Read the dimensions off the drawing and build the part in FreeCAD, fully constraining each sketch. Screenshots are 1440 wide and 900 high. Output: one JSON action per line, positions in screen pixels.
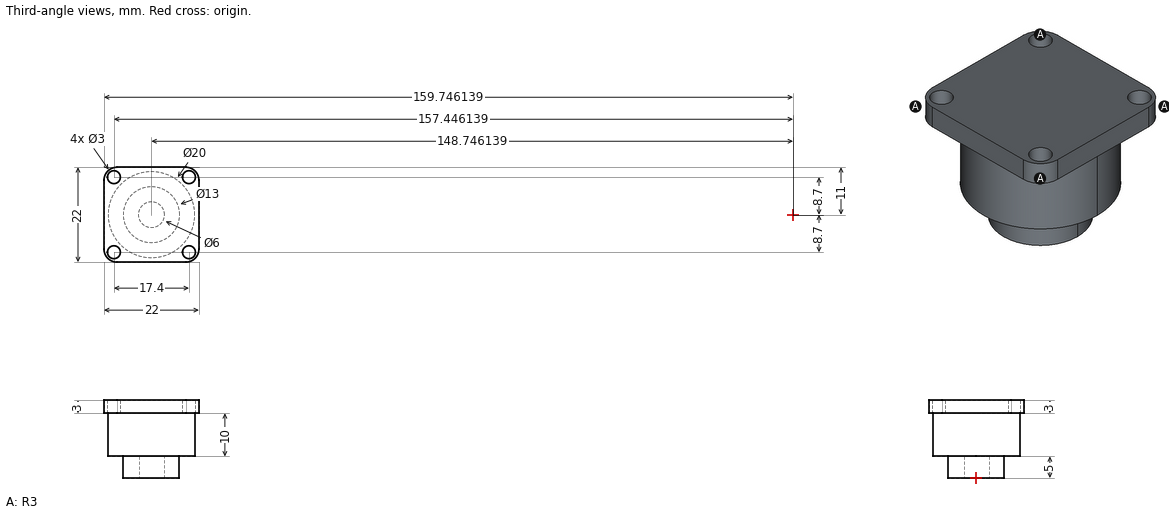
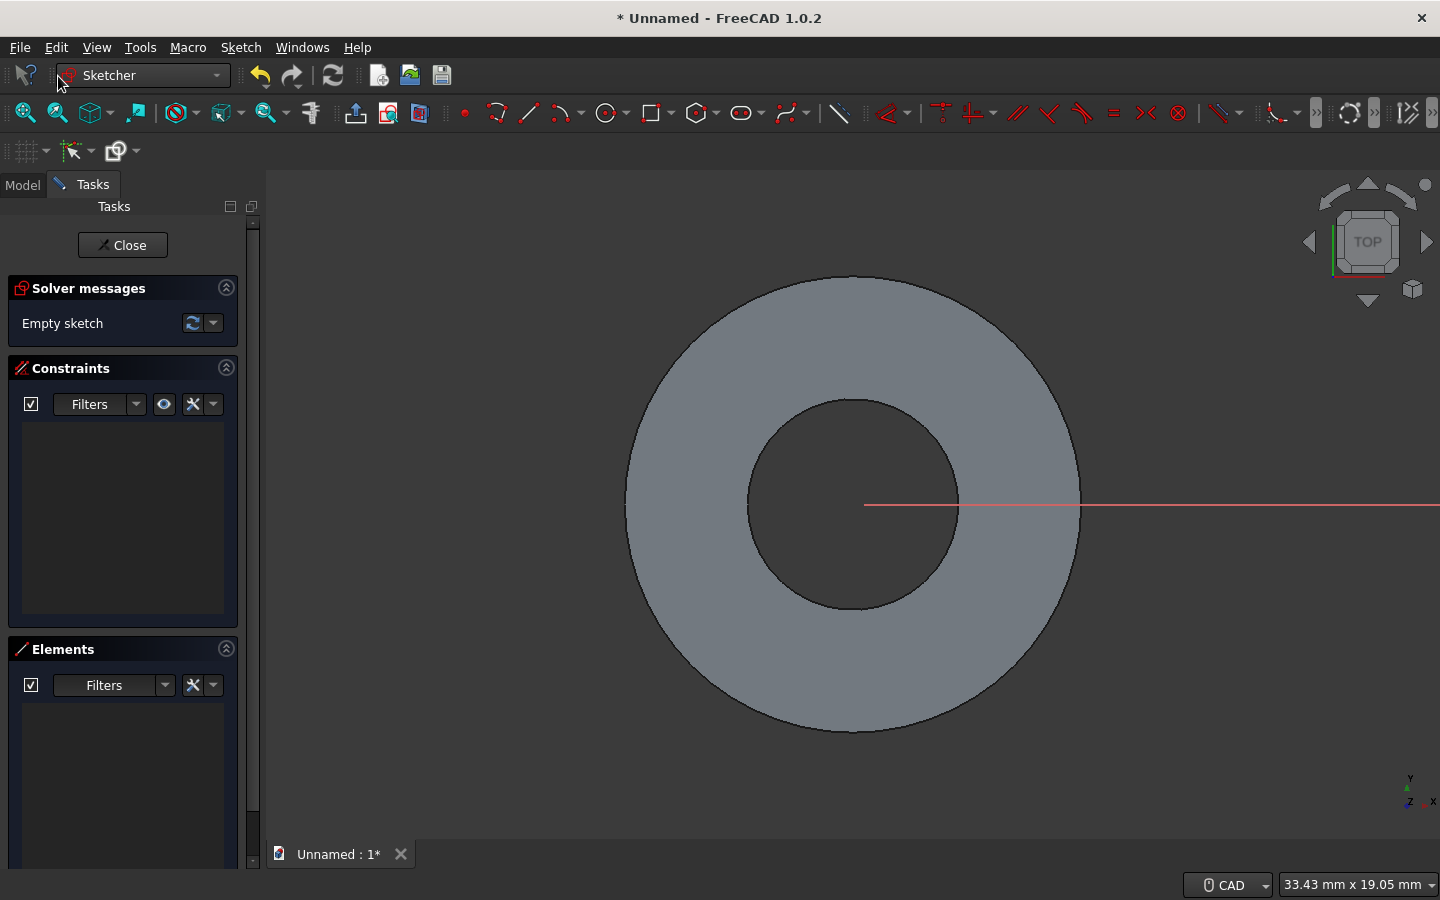
{"action": "scroll", "coordinate": [645, 504], "scroll_direction": "down", "scroll_amount": 2}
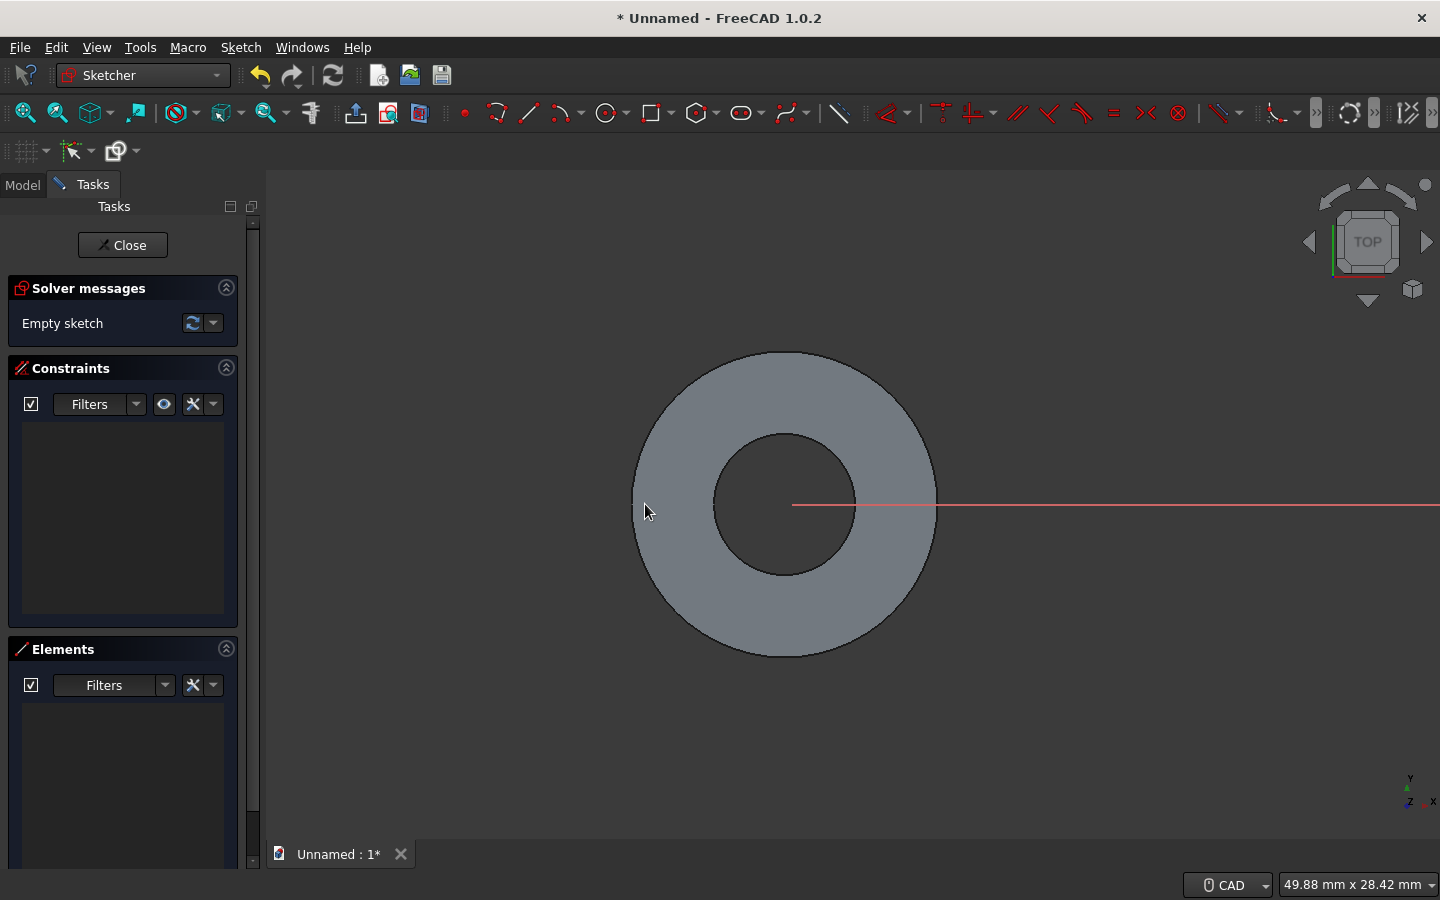
{"action": "left_click", "coordinate": [606, 114]}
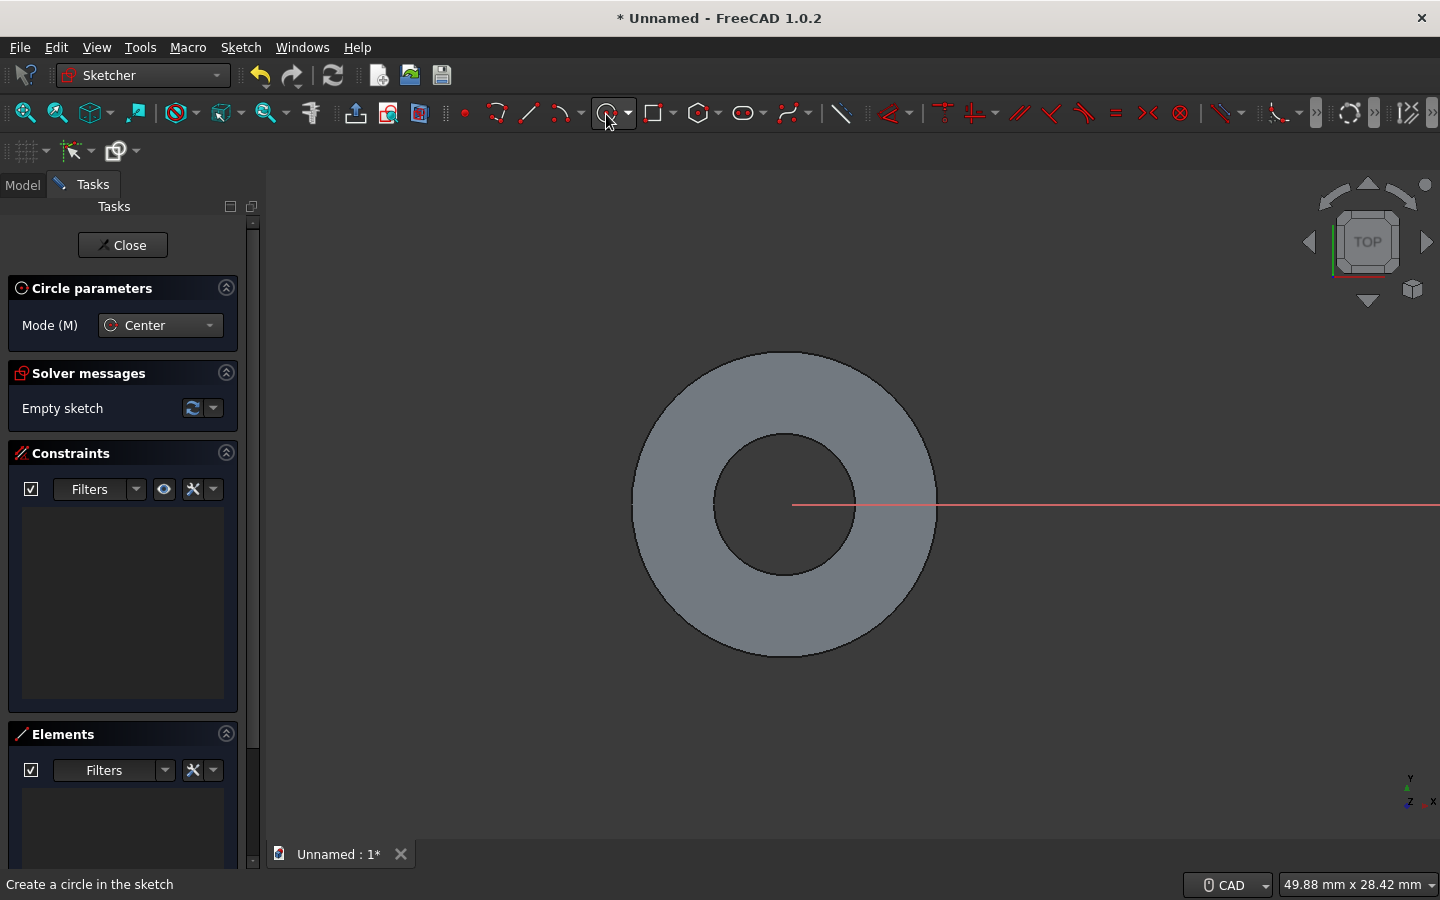
{"action": "left_click", "coordinate": [785, 504]}
{"action": "mouse_move", "coordinate": [951, 338]}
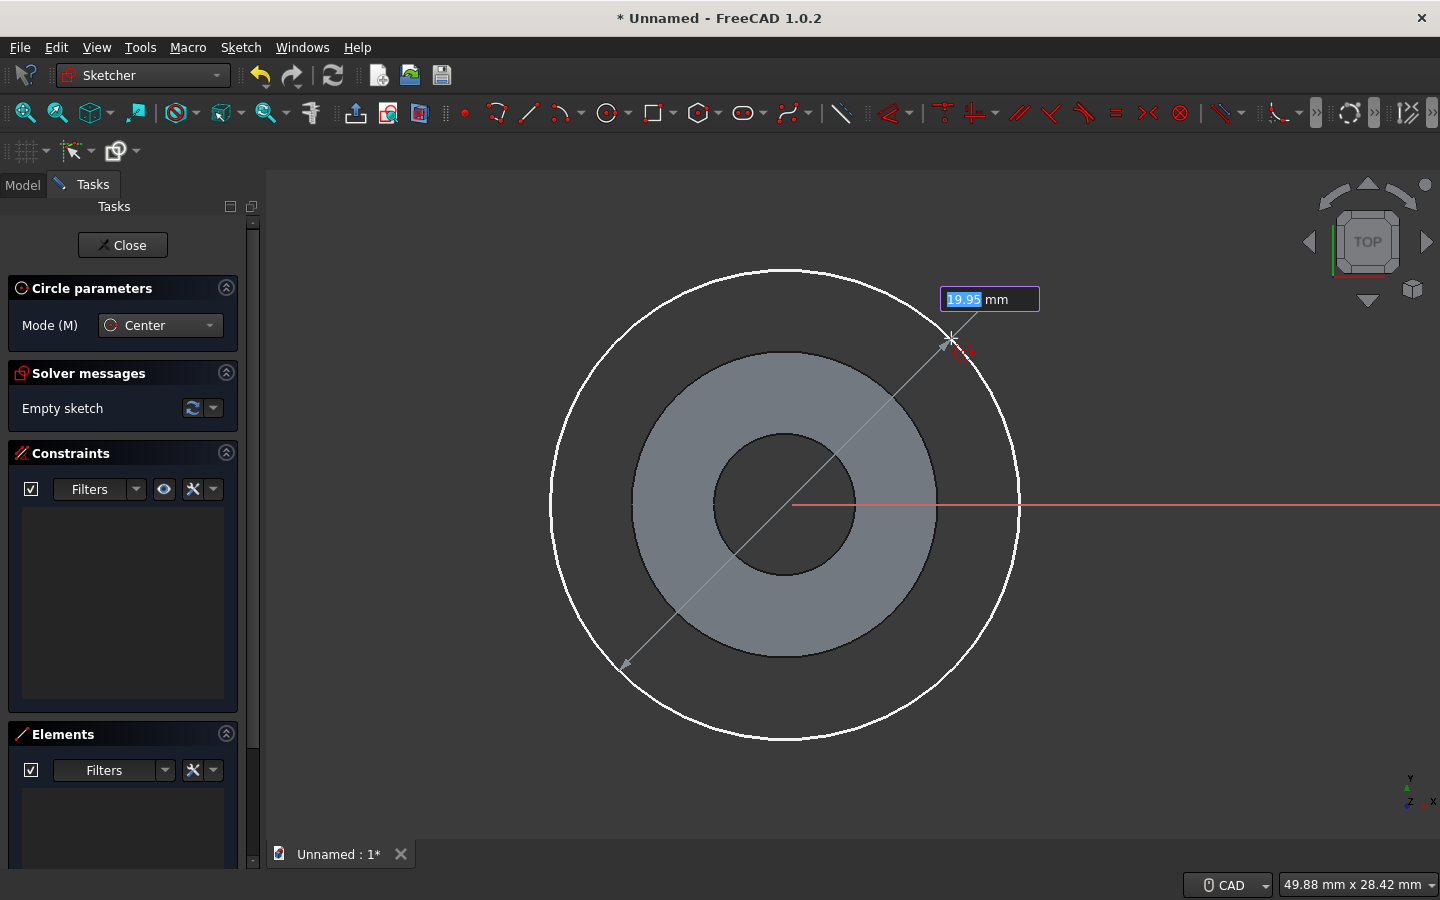
{"action": "type", "text": "20"}
{"action": "key", "text": "Return"}
{"action": "key", "text": "Escape"}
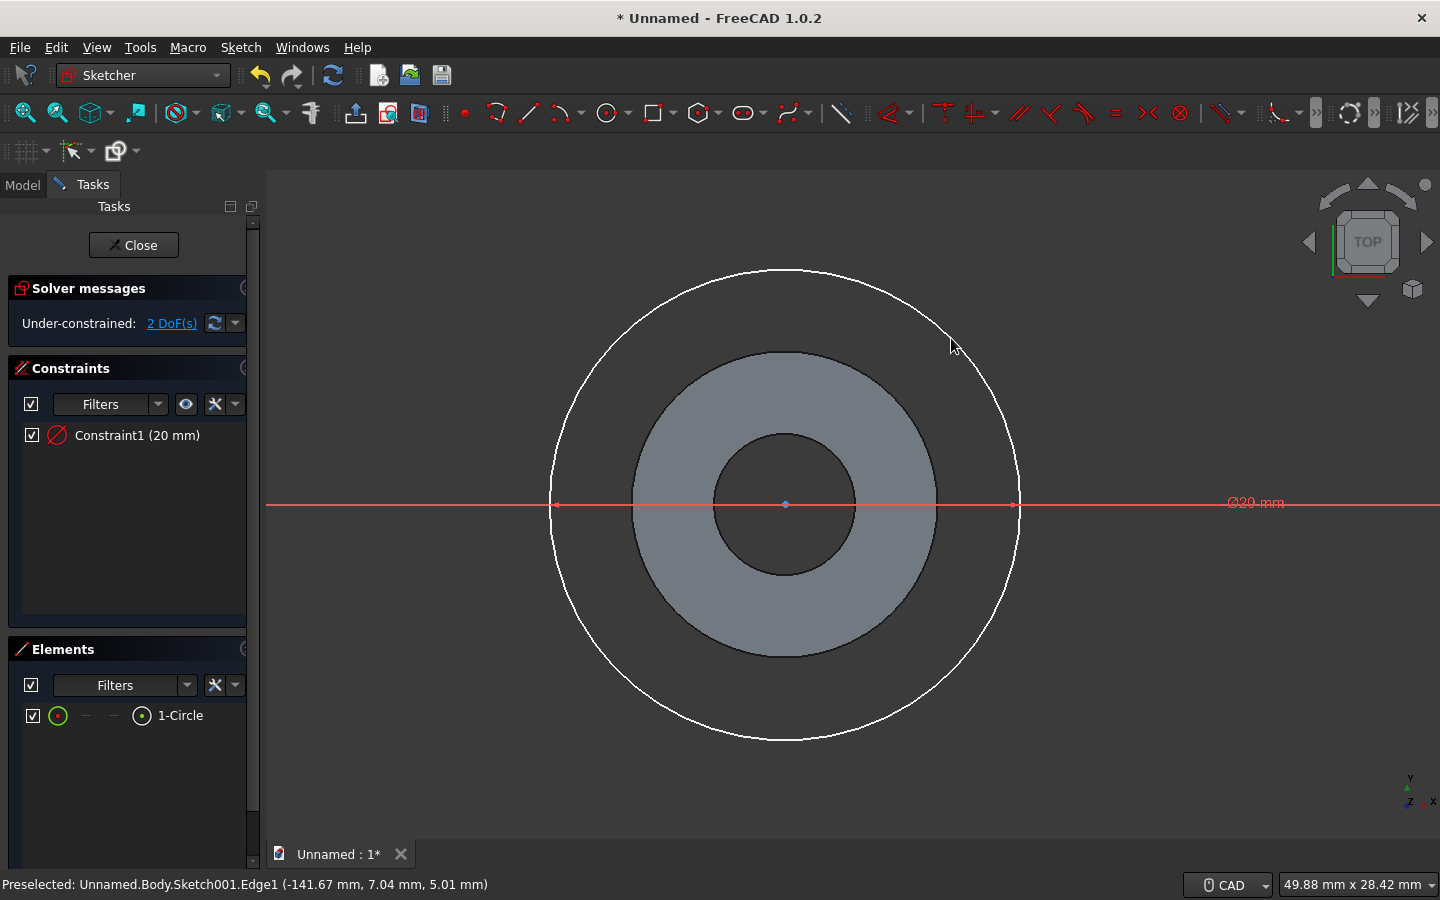
{"action": "left_click", "coordinate": [785, 505]}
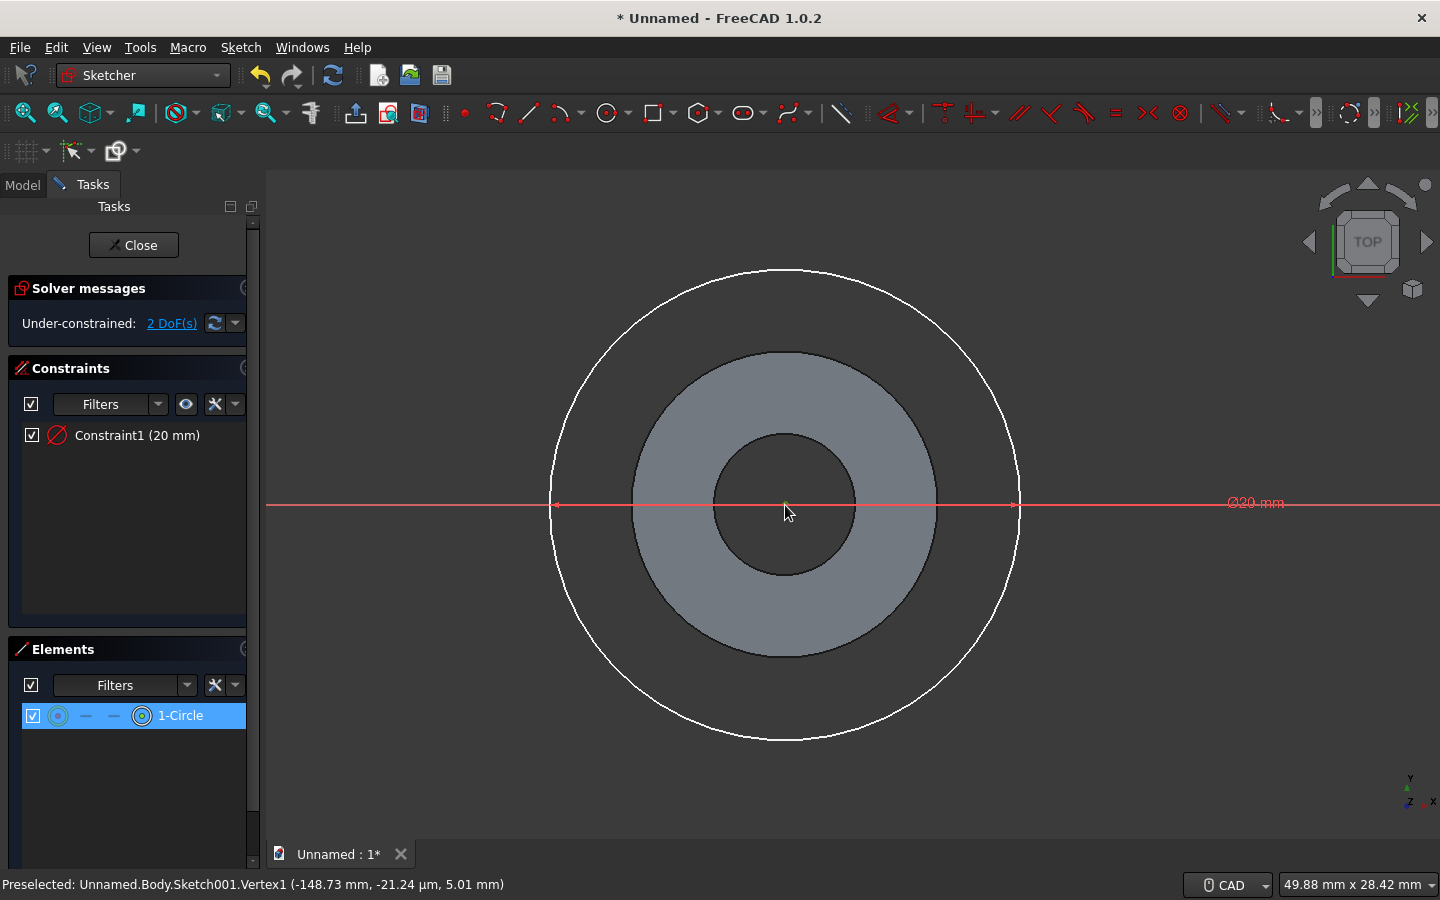
{"action": "left_click", "coordinate": [364, 504]}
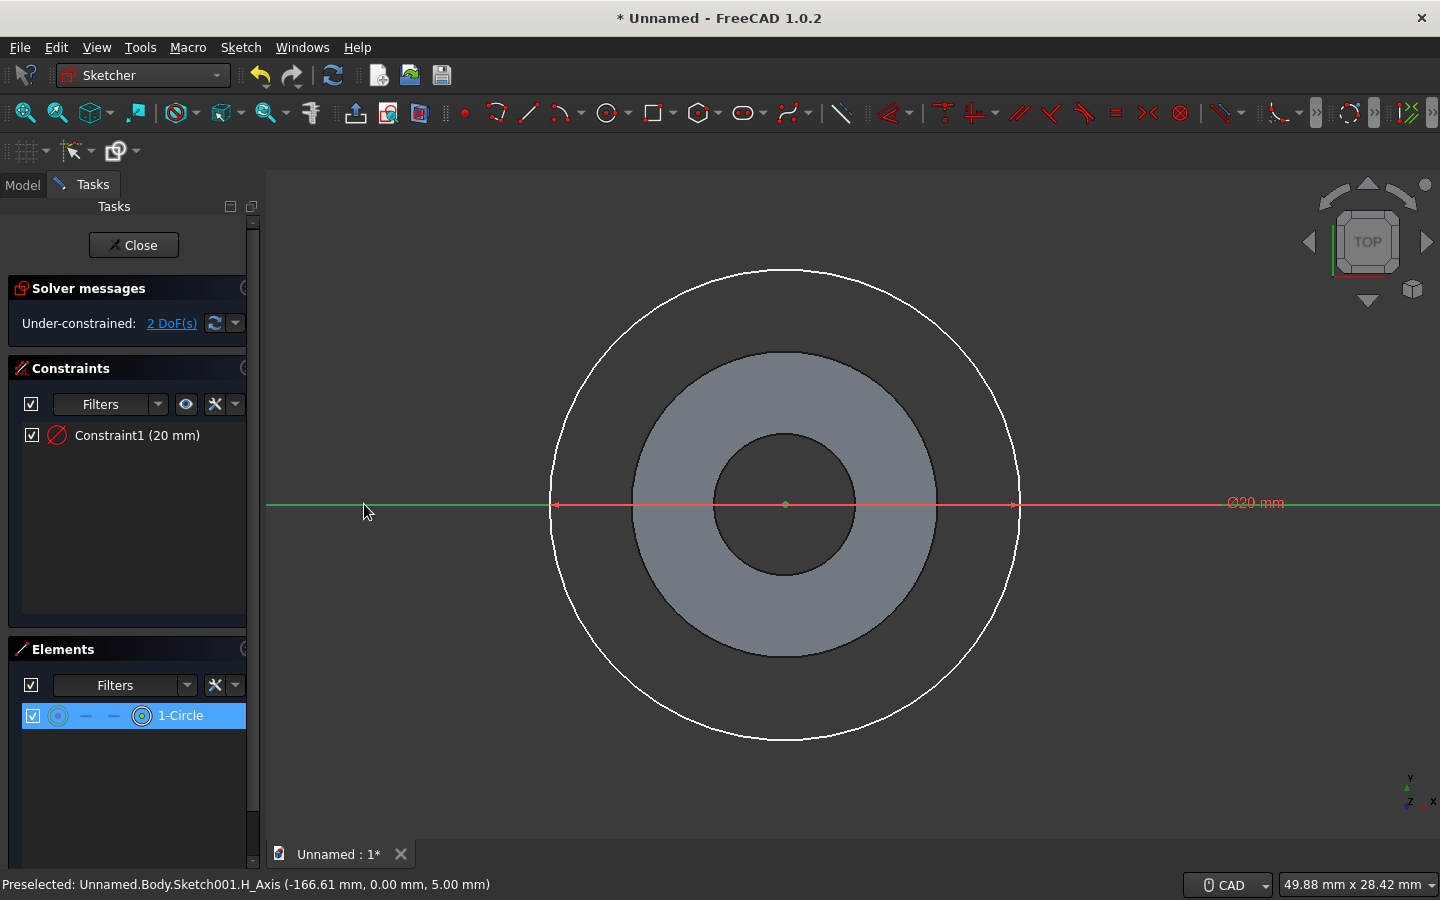
{"action": "left_click", "coordinate": [944, 114]}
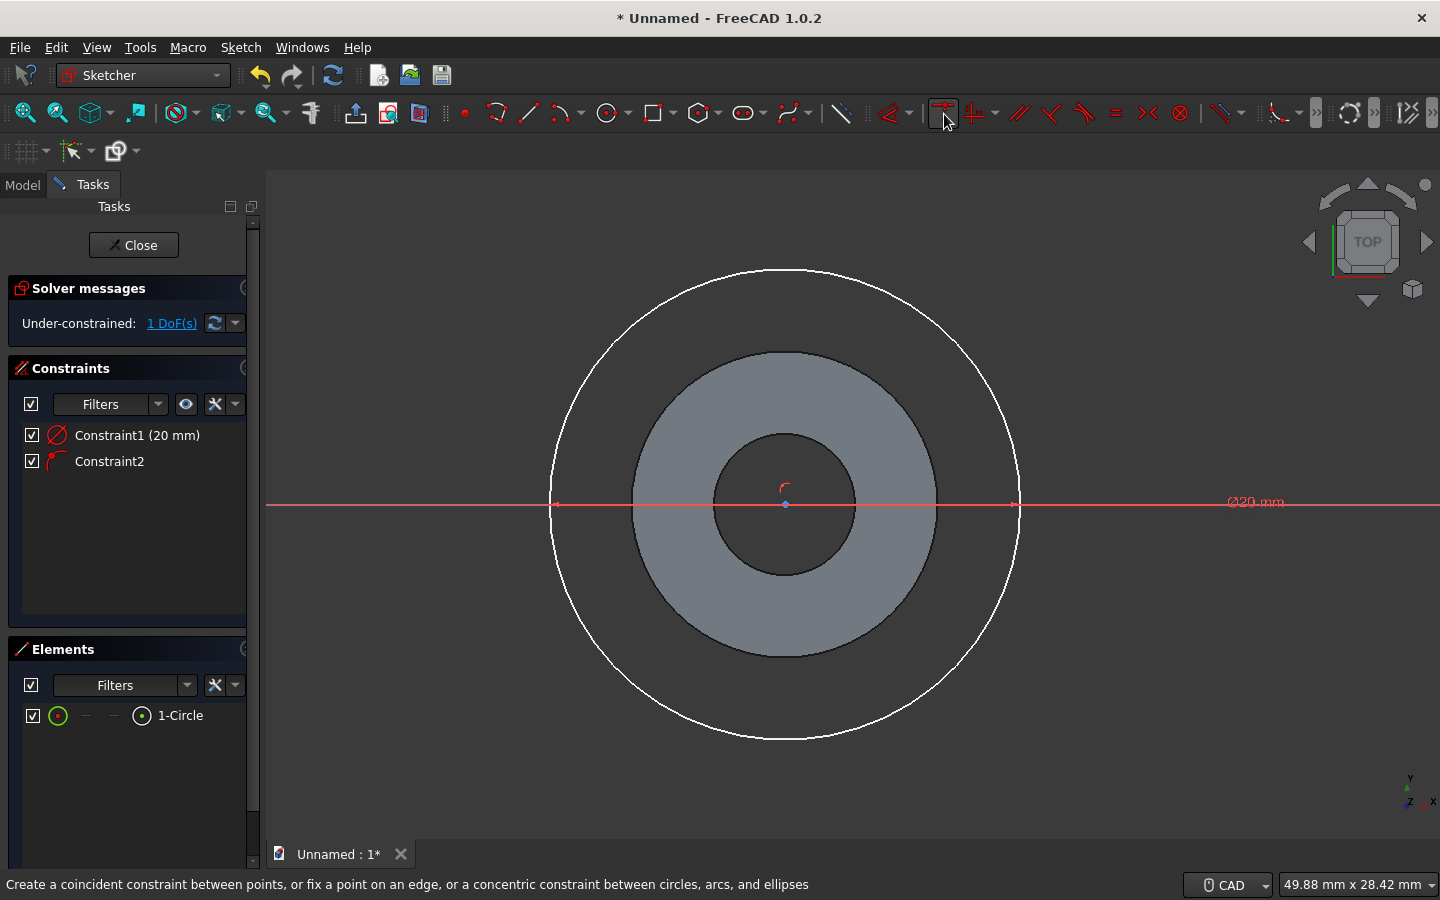
{"action": "left_click", "coordinate": [888, 114]}